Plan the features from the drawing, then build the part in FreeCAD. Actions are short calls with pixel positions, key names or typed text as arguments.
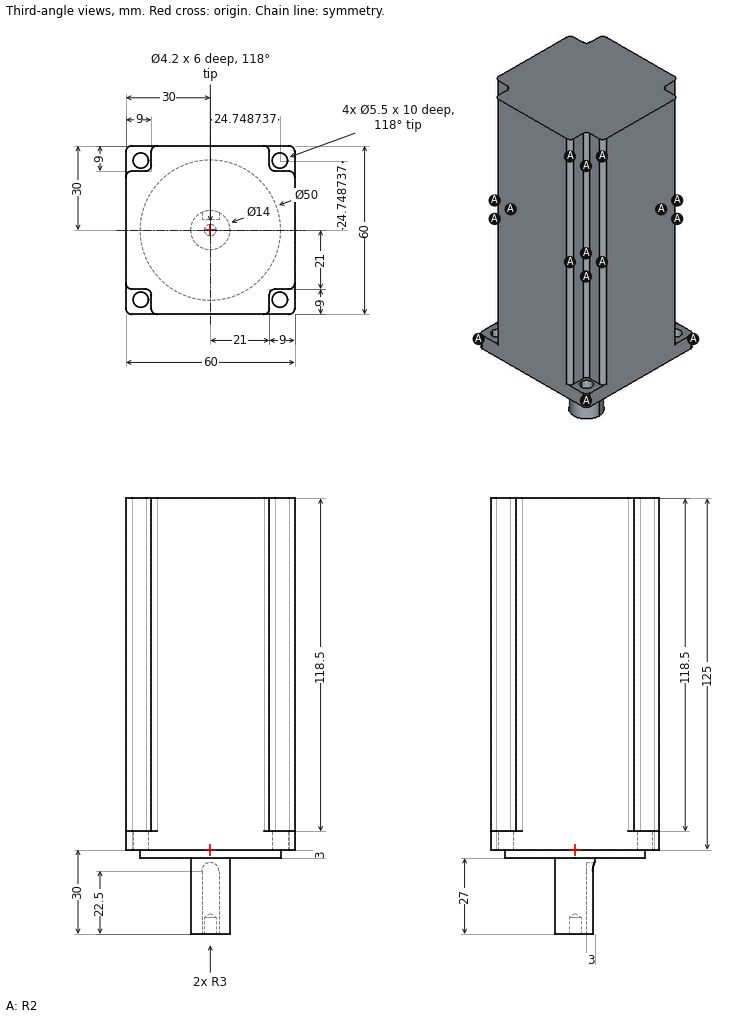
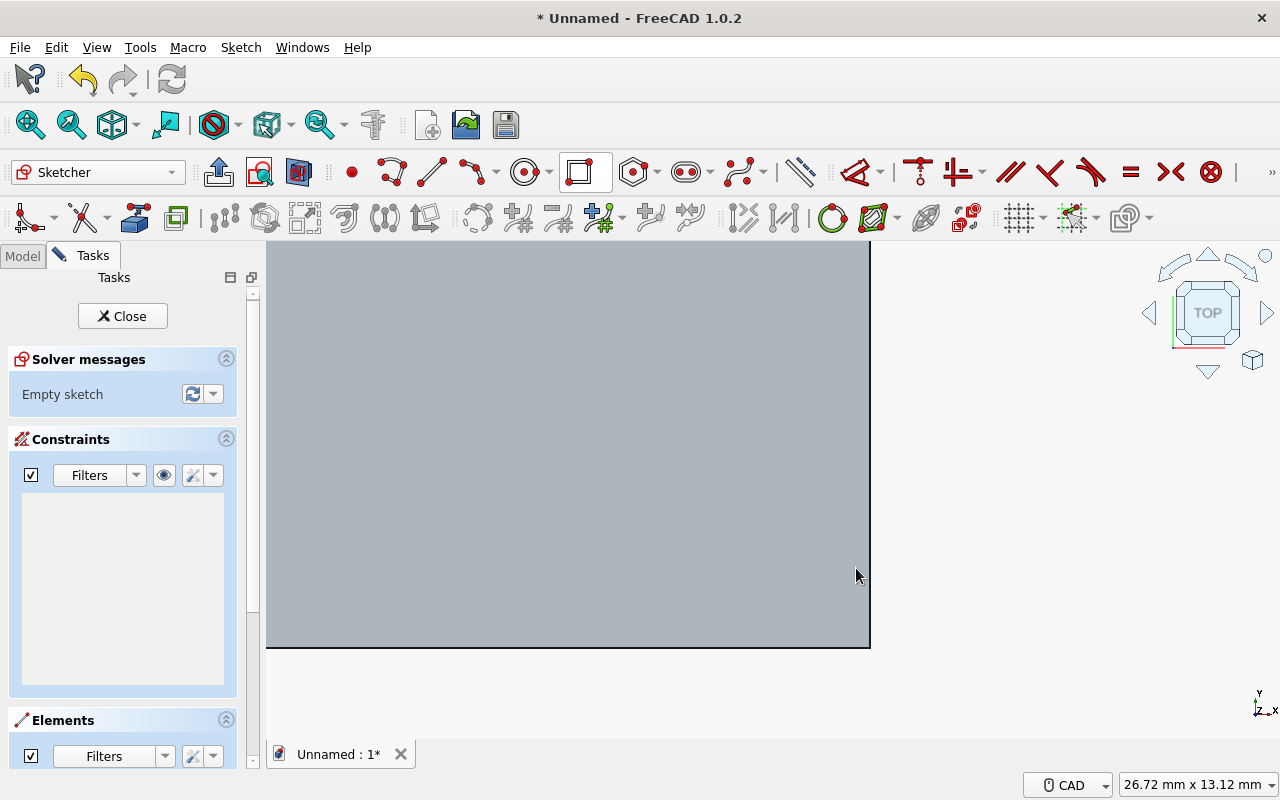
click(580, 172)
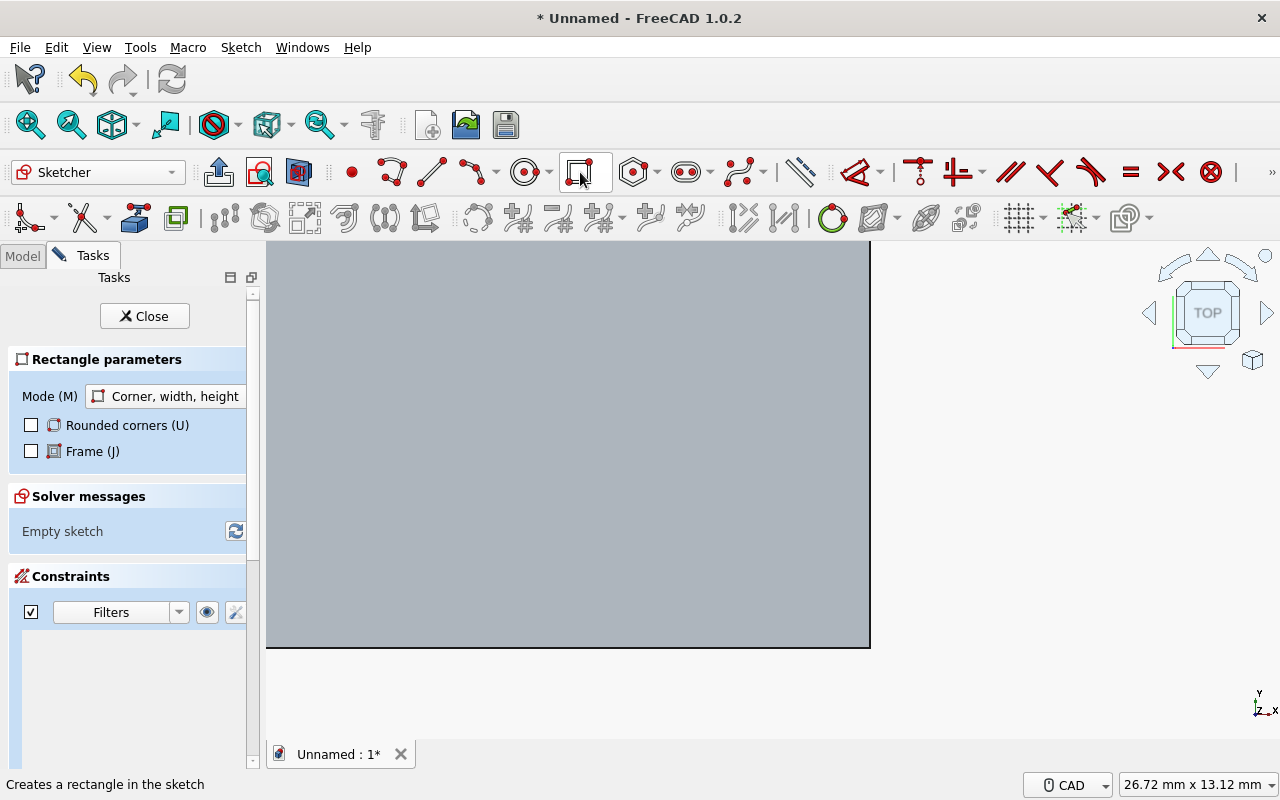
click(528, 306)
move(870, 648)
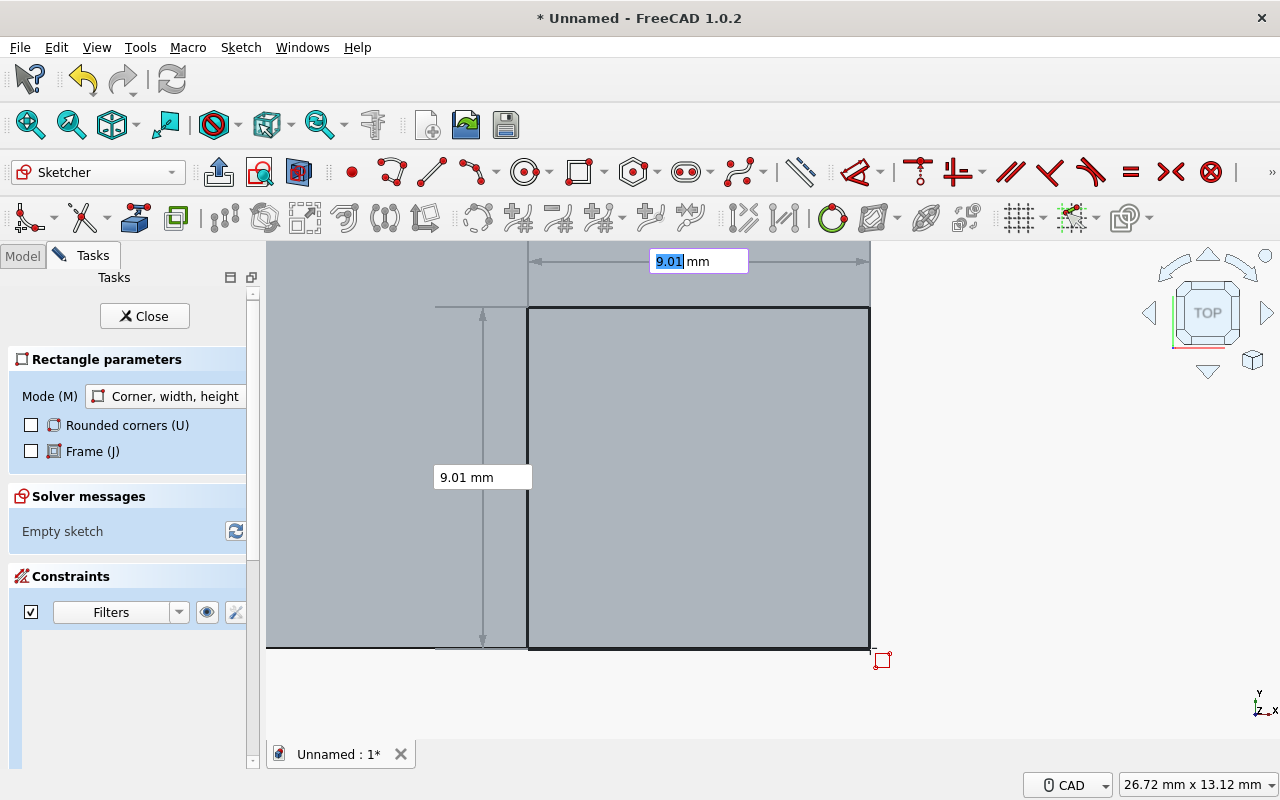
text(9)
key(Tab)
text(9)
key(Return)
key(Escape)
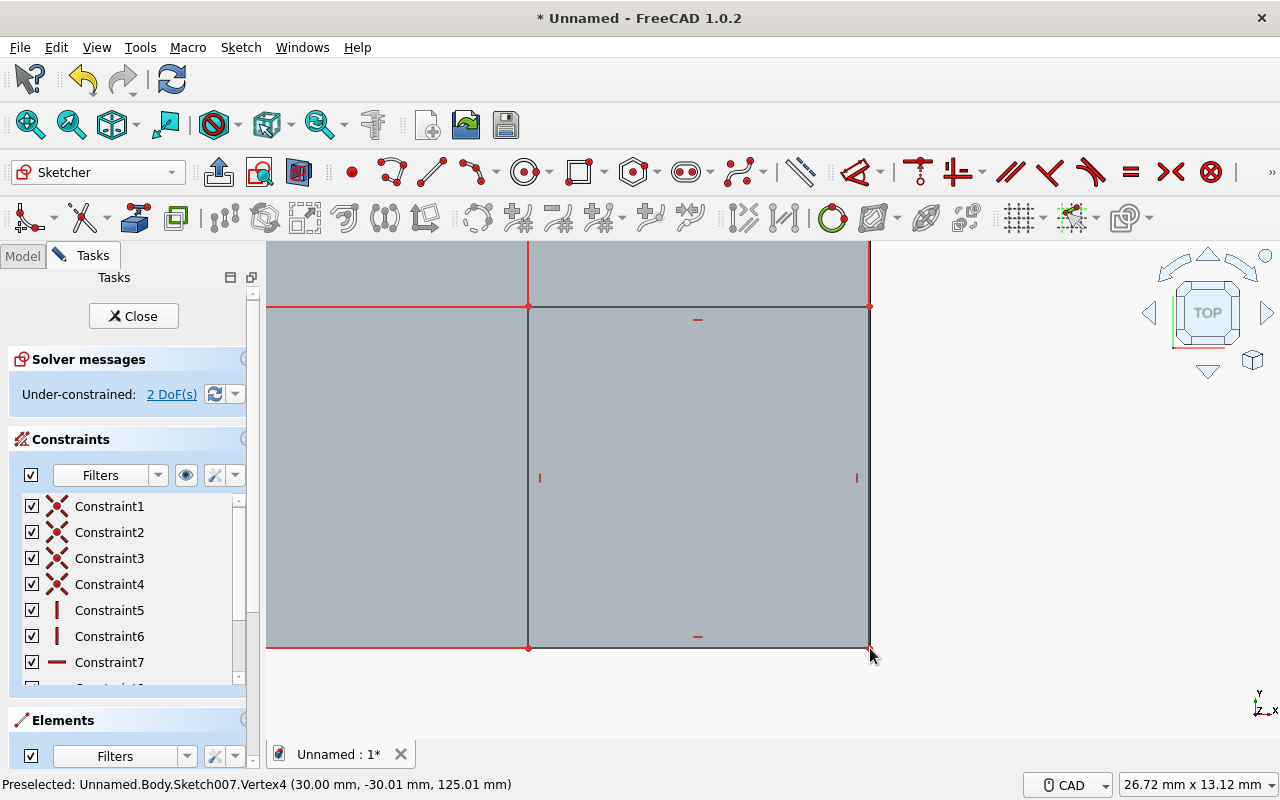
click(856, 172)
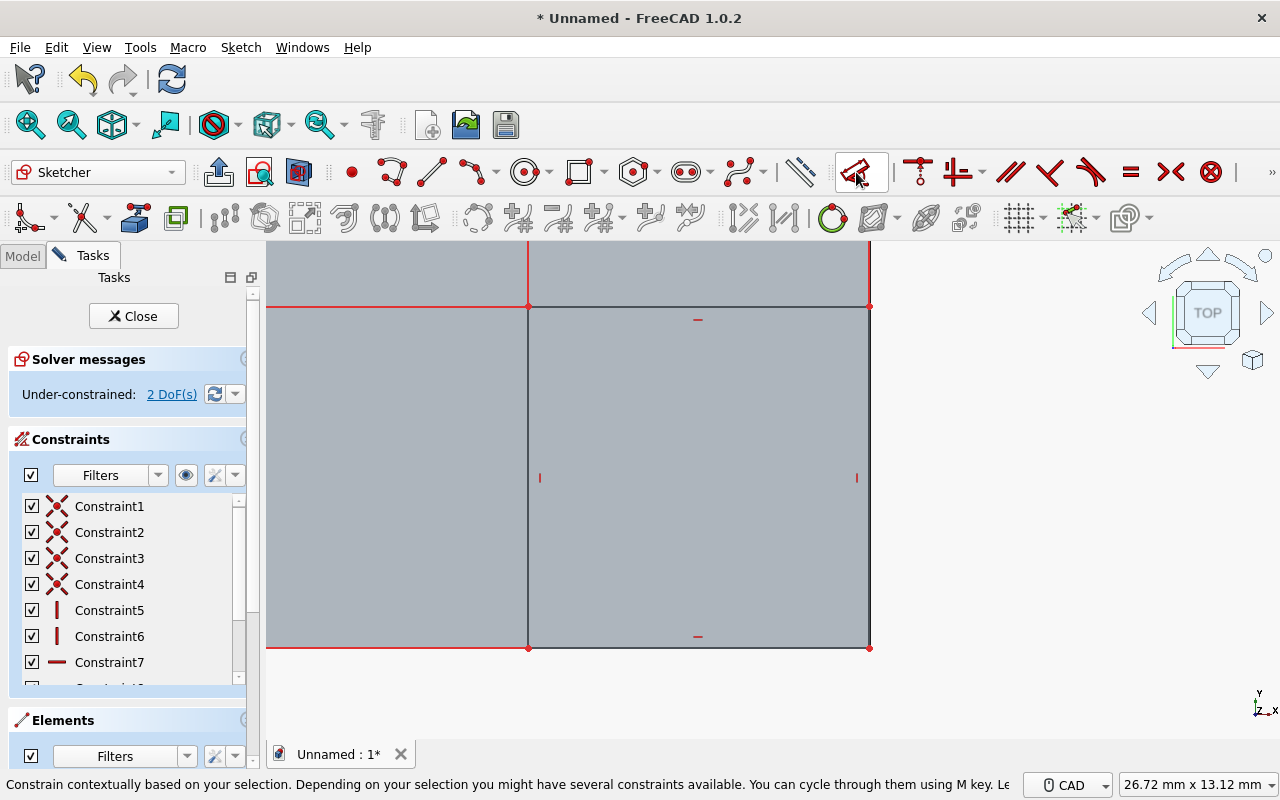
click(528, 307)
click(411, 341)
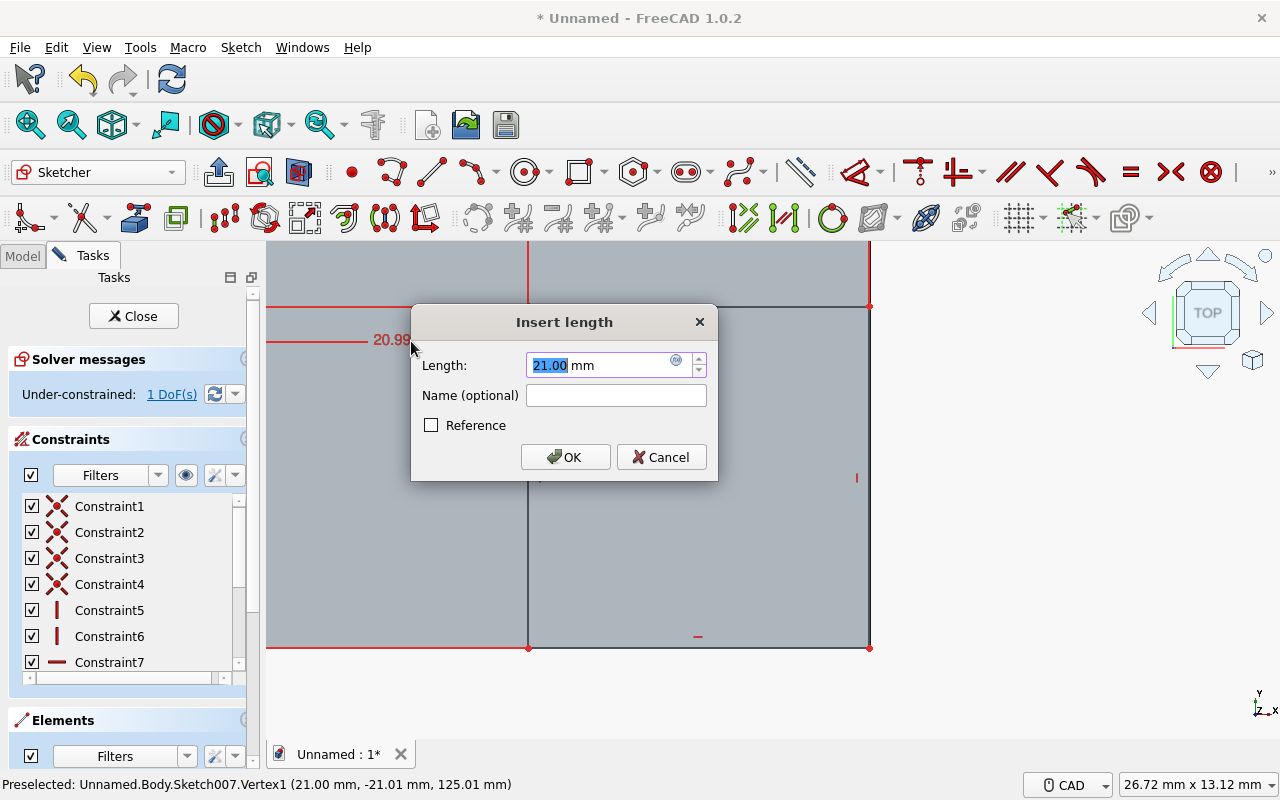
text(21)
key(Return)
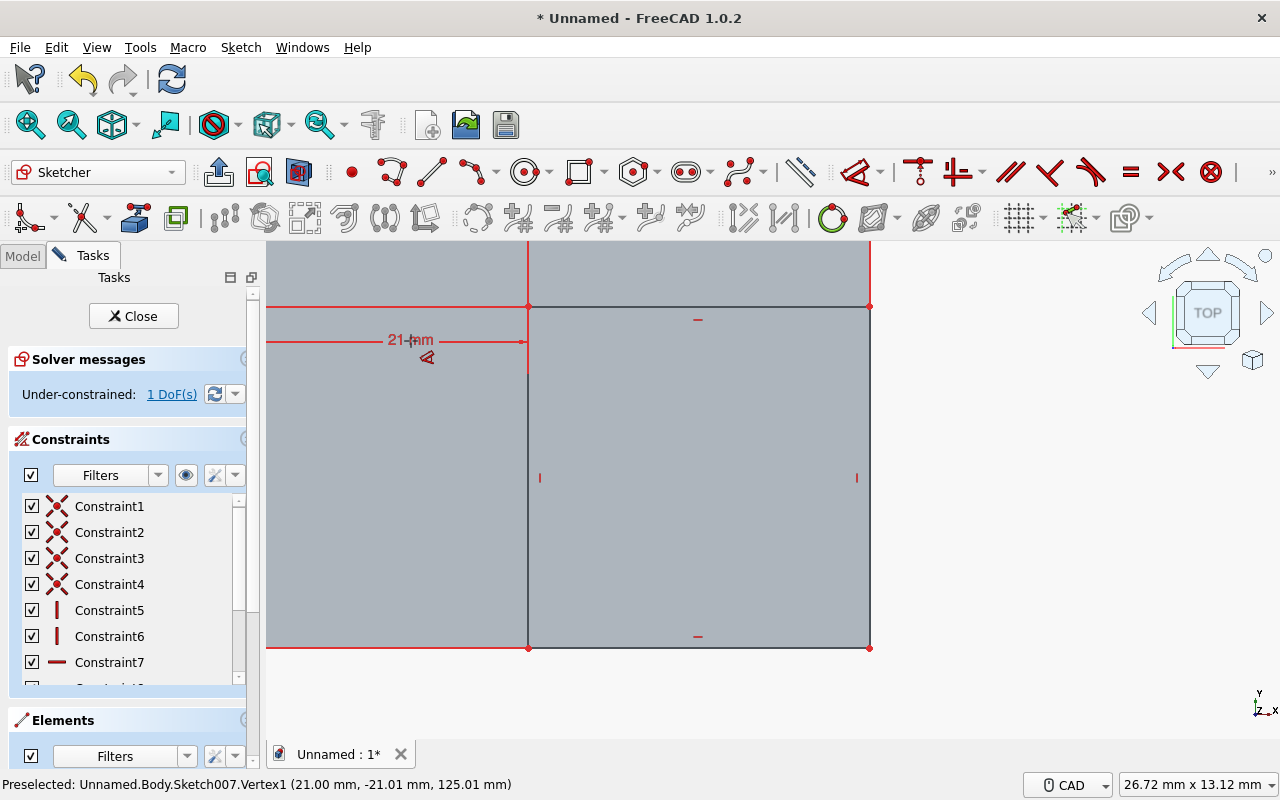
click(528, 307)
click(562, 288)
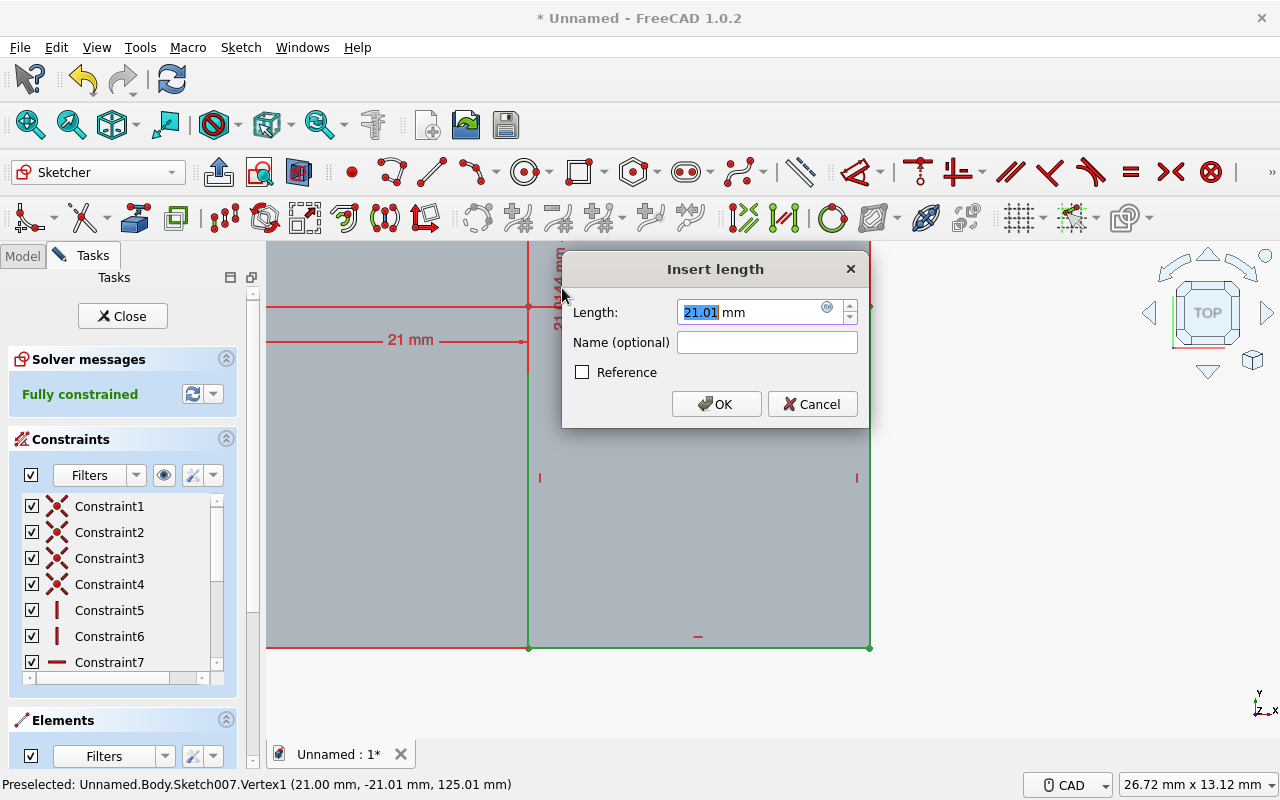
text(21)
key(Return)
key(Escape)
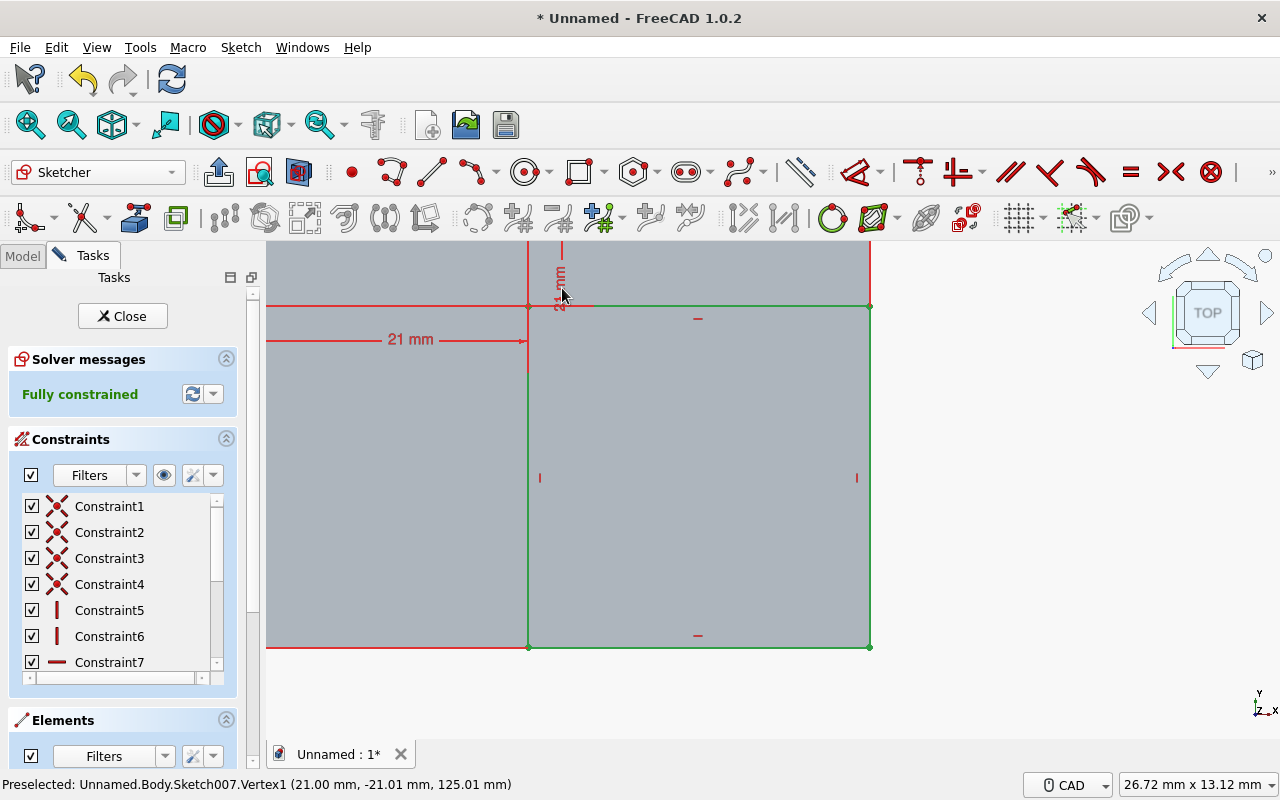
click(123, 316)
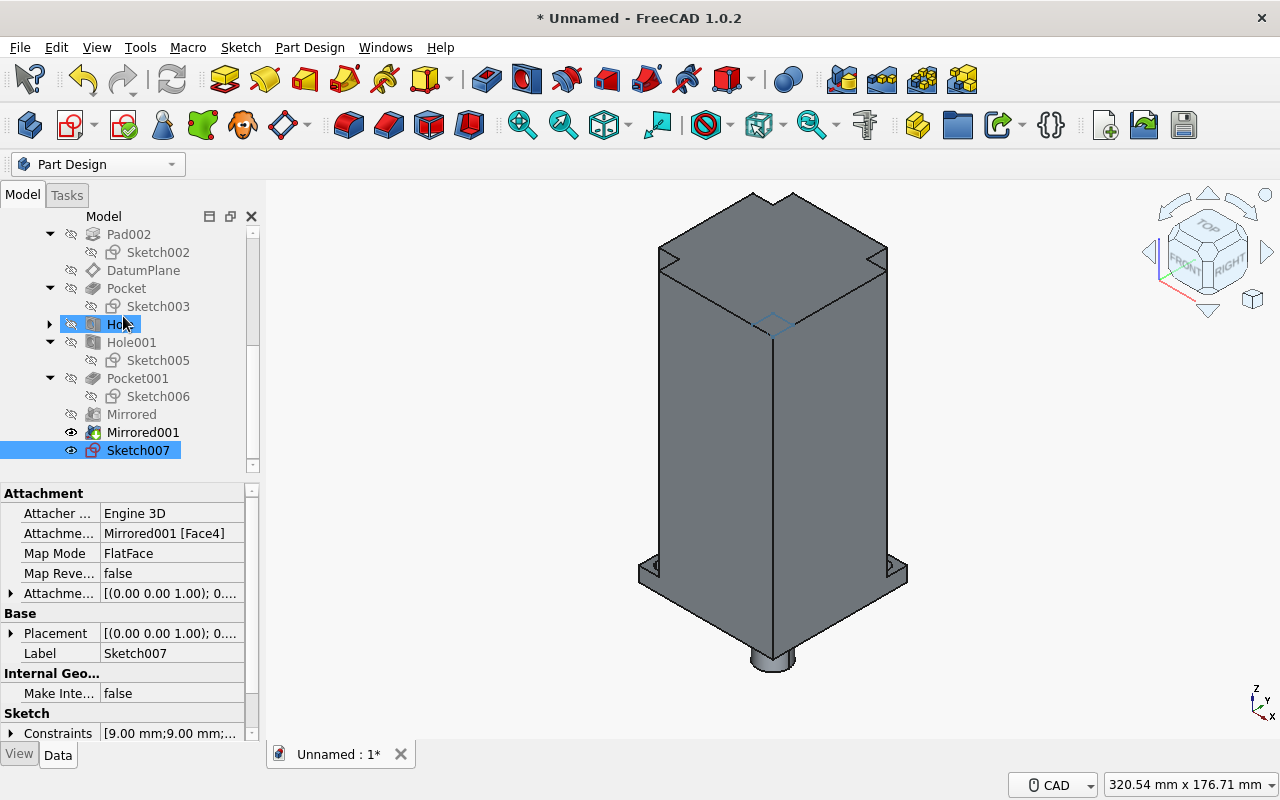
click(488, 80)